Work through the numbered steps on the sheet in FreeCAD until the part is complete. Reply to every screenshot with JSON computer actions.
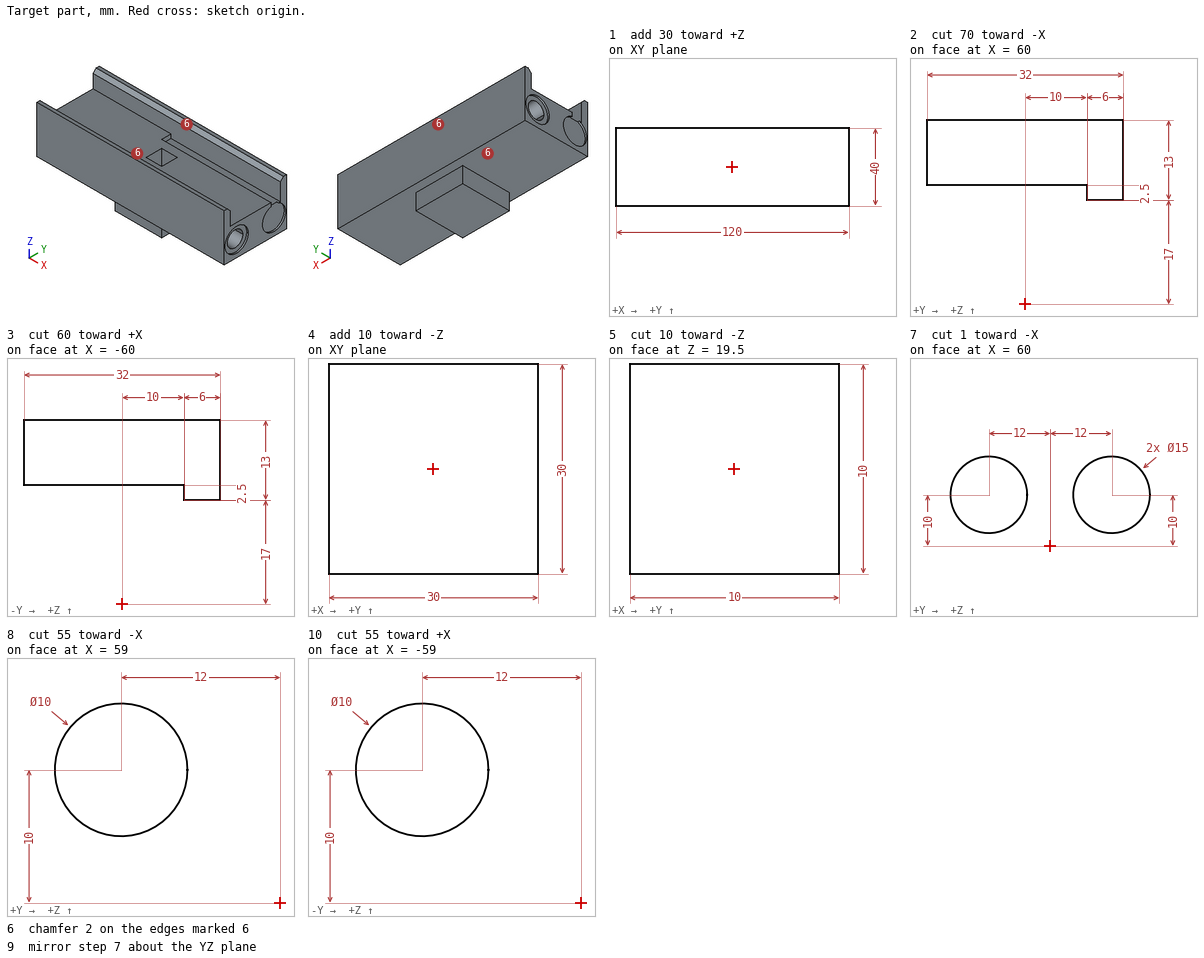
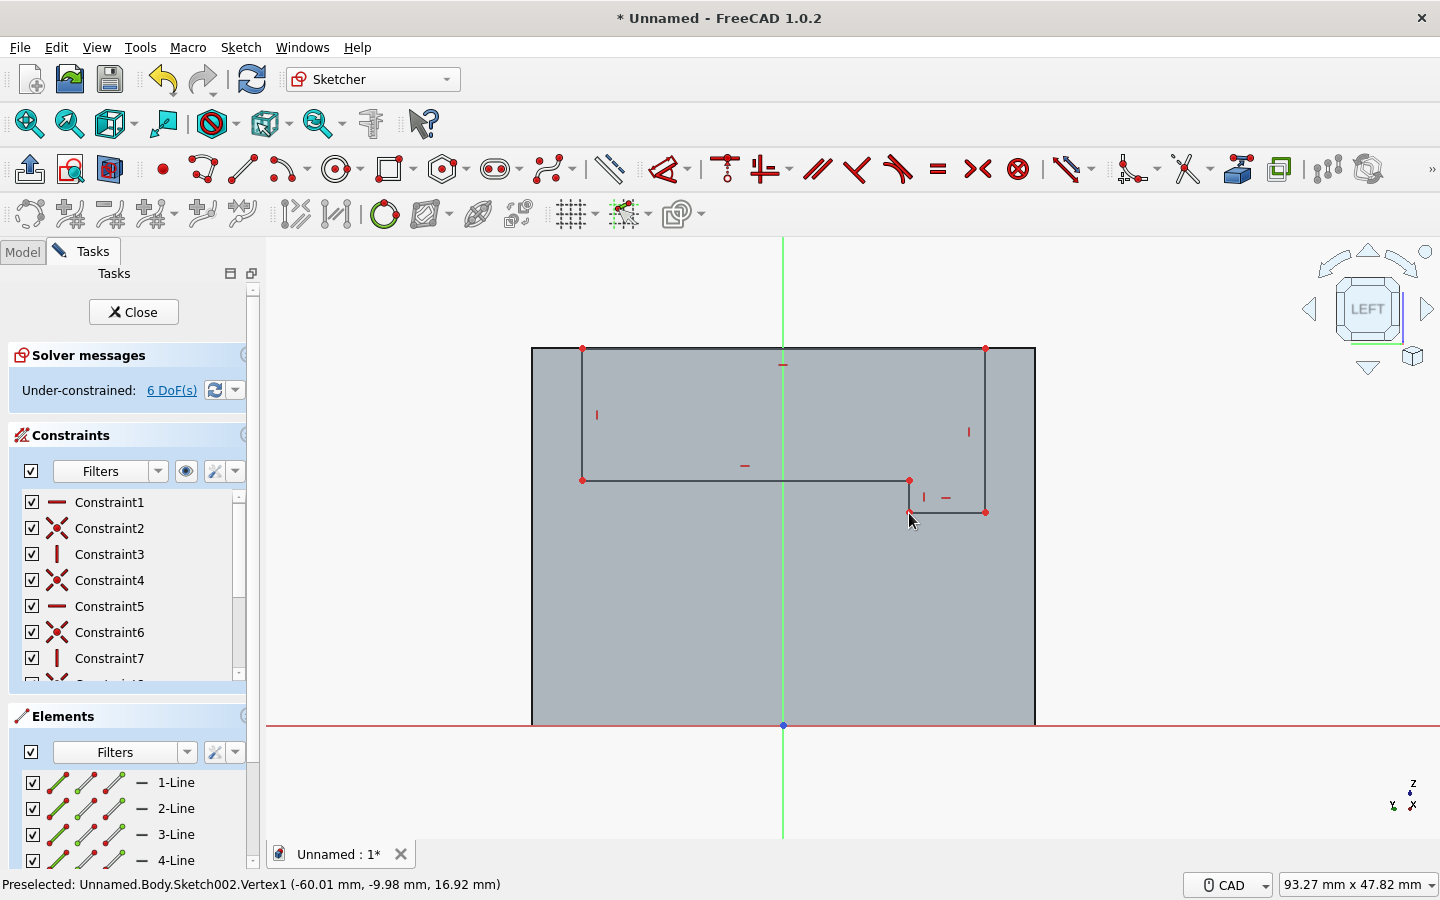
{"action": "left_click", "coordinate": [664, 170]}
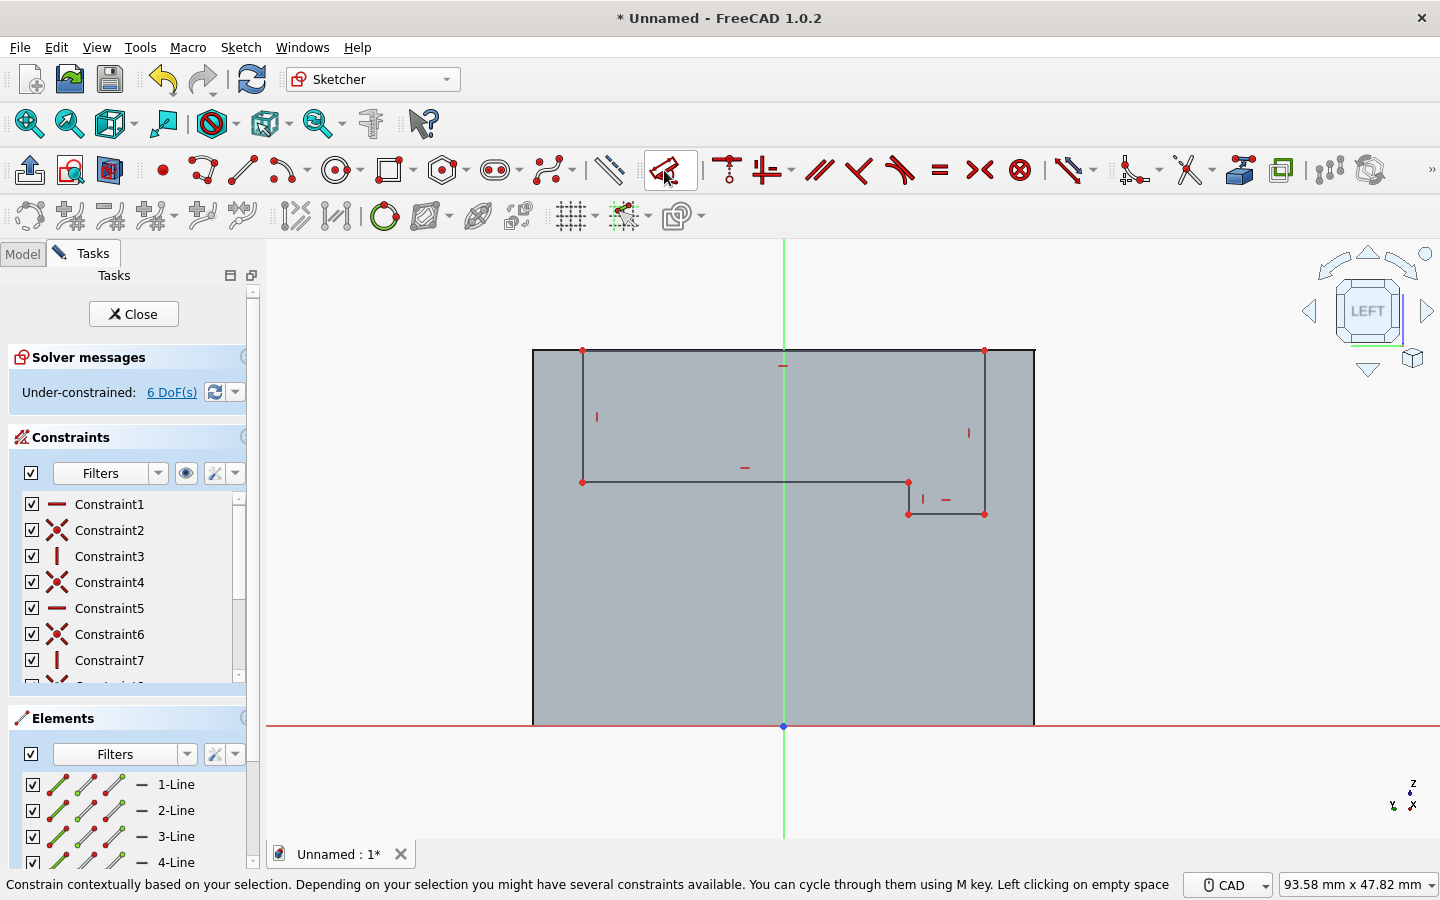
{"action": "left_click", "coordinate": [932, 514]}
{"action": "left_click", "coordinate": [947, 480]}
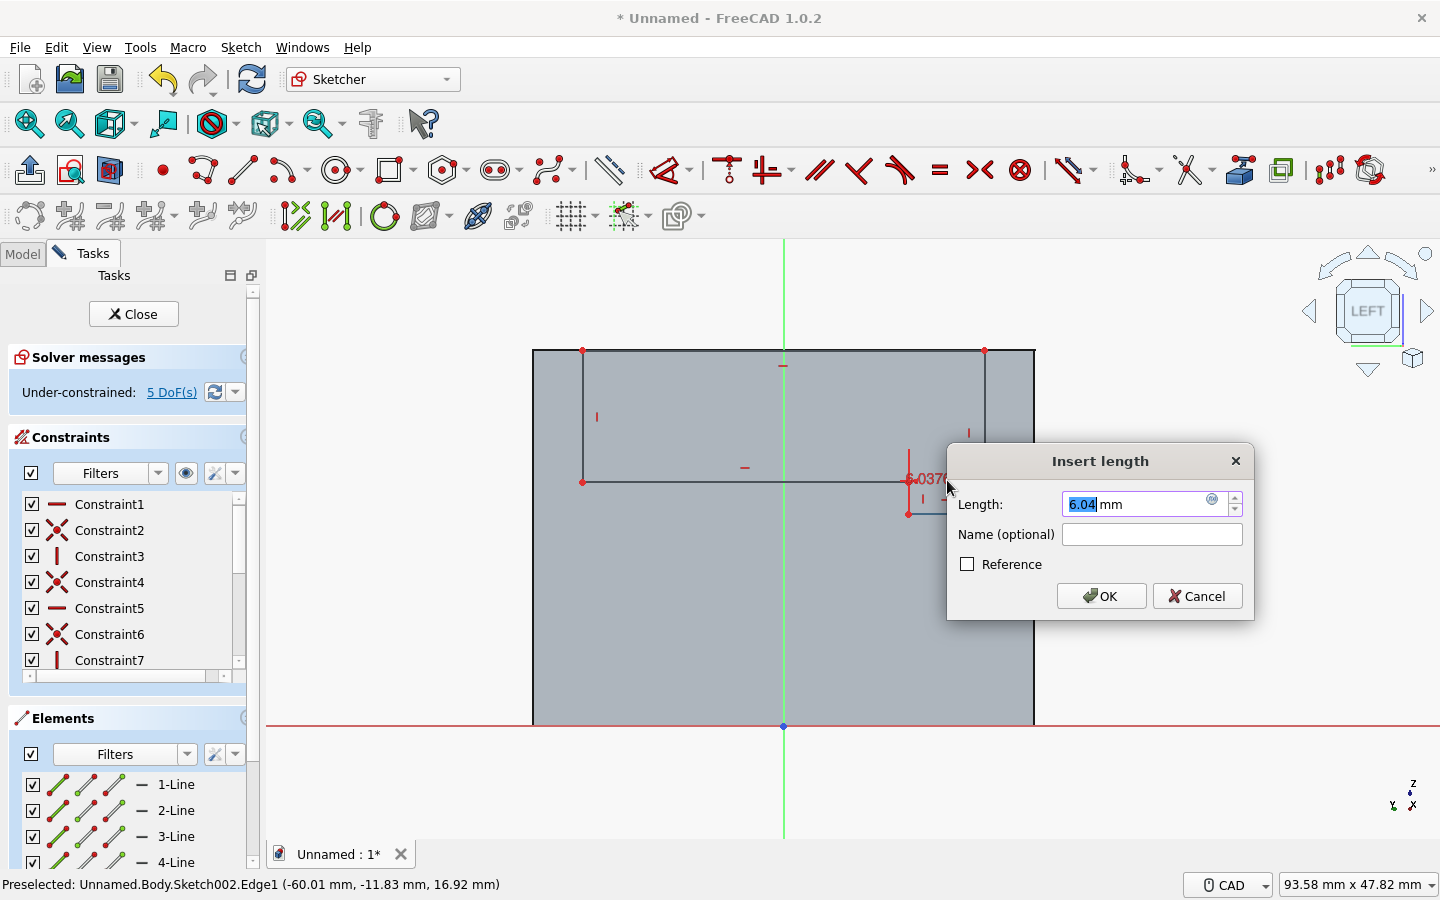
{"action": "type", "text": "6"}
{"action": "key", "text": "Return"}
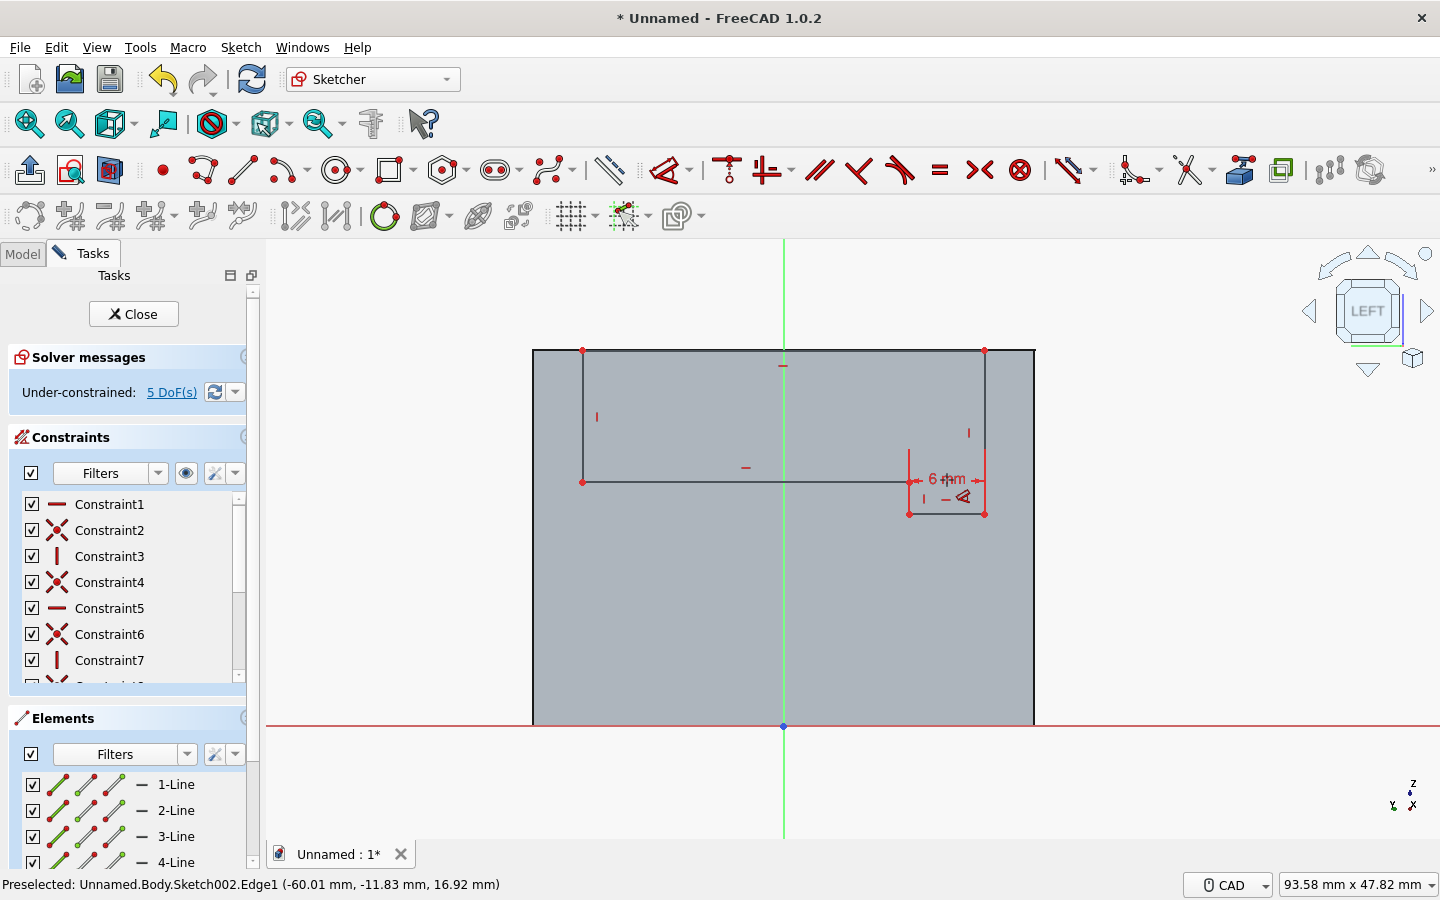
{"action": "left_click", "coordinate": [985, 465]}
{"action": "left_click", "coordinate": [1019, 432]}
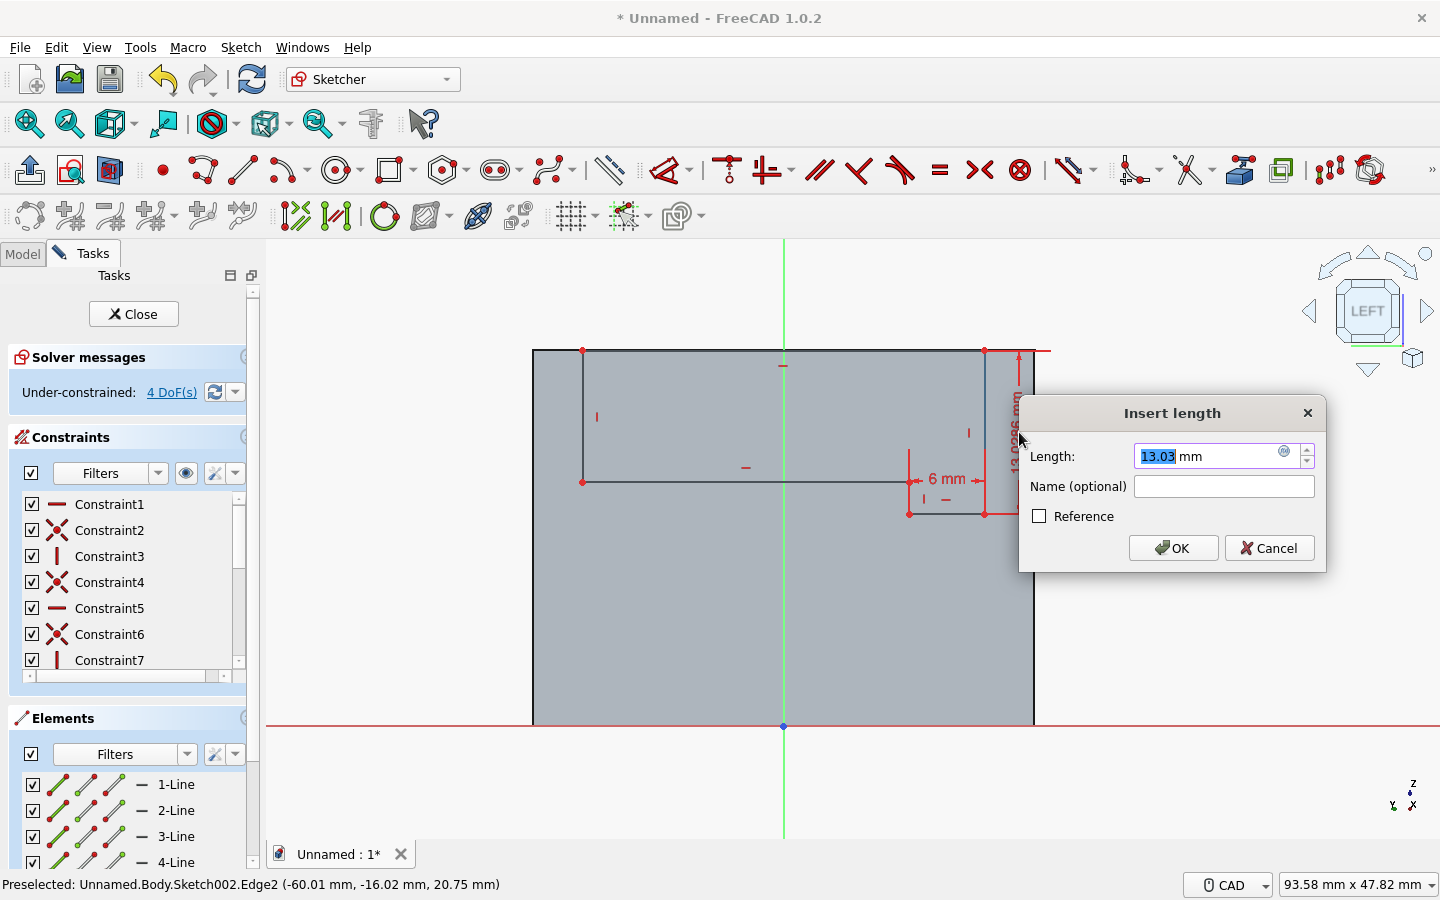
{"action": "type", "text": "13"}
{"action": "key", "text": "Return"}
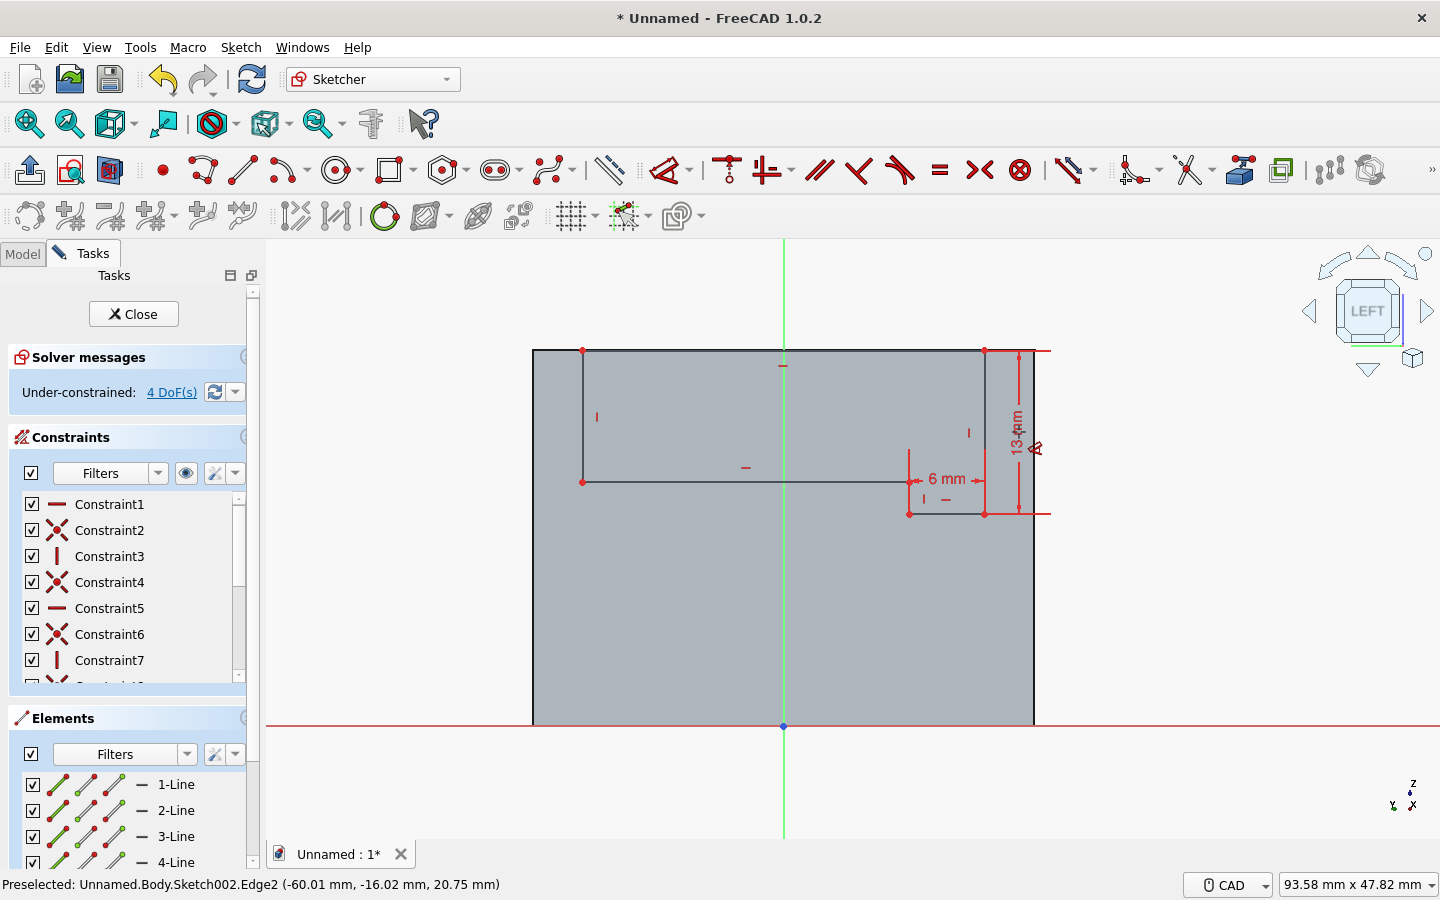
{"action": "left_click", "coordinate": [864, 351]}
{"action": "left_click", "coordinate": [691, 317]}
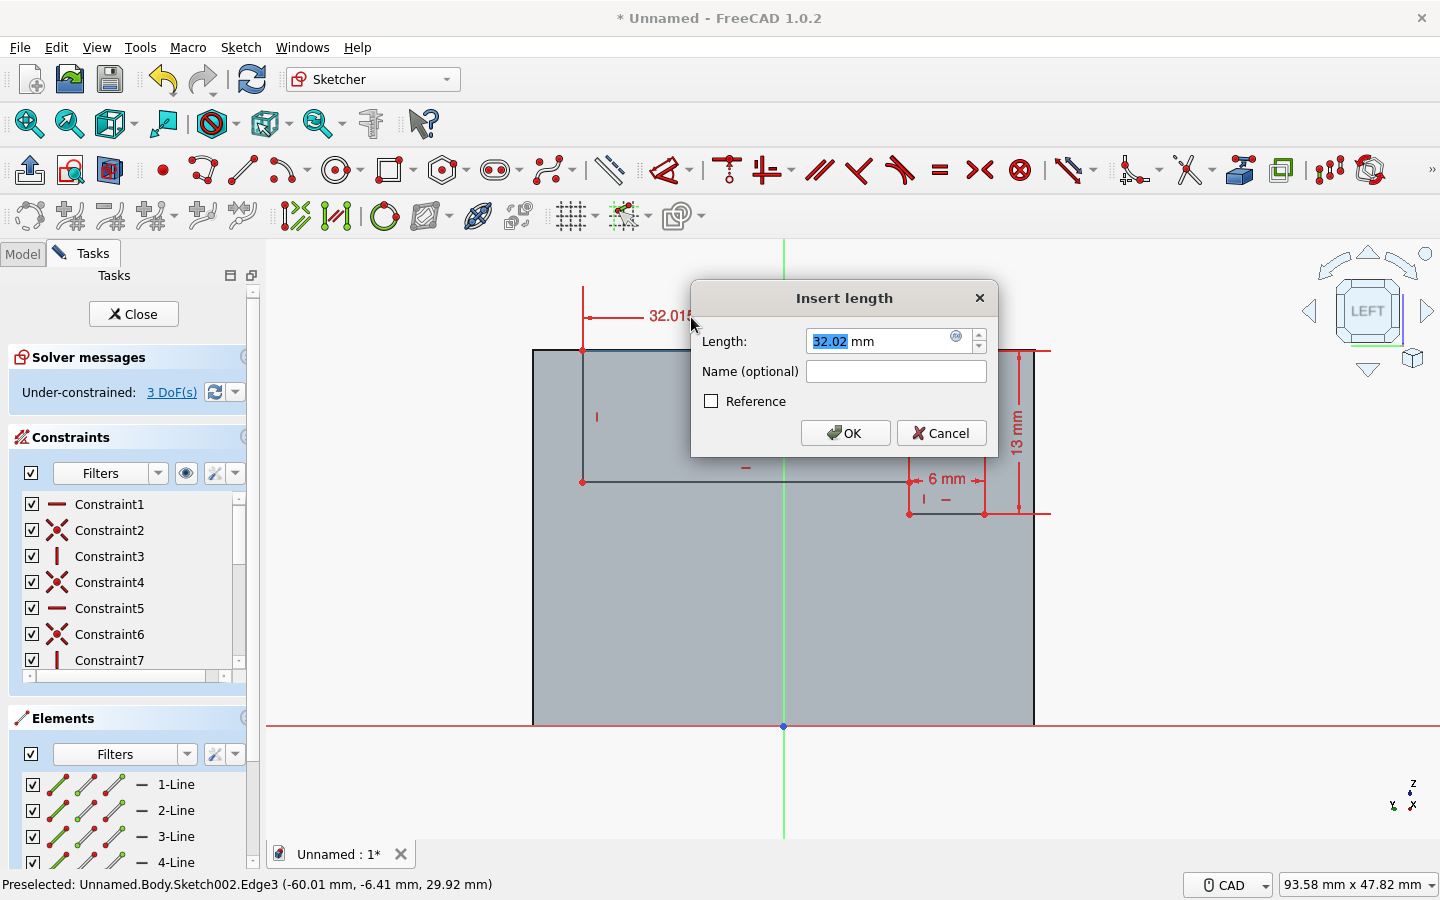
{"action": "type", "text": "32"}
{"action": "key", "text": "Return"}